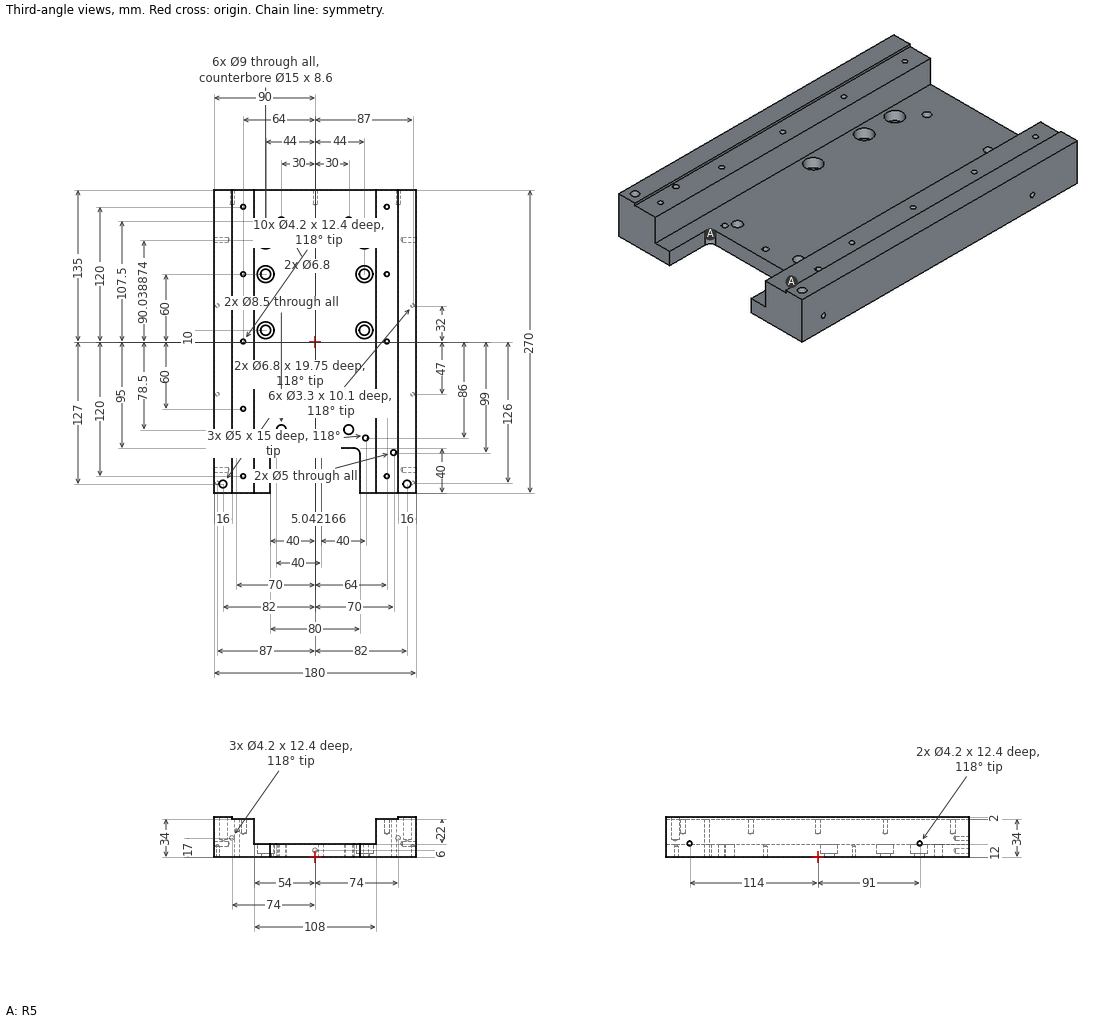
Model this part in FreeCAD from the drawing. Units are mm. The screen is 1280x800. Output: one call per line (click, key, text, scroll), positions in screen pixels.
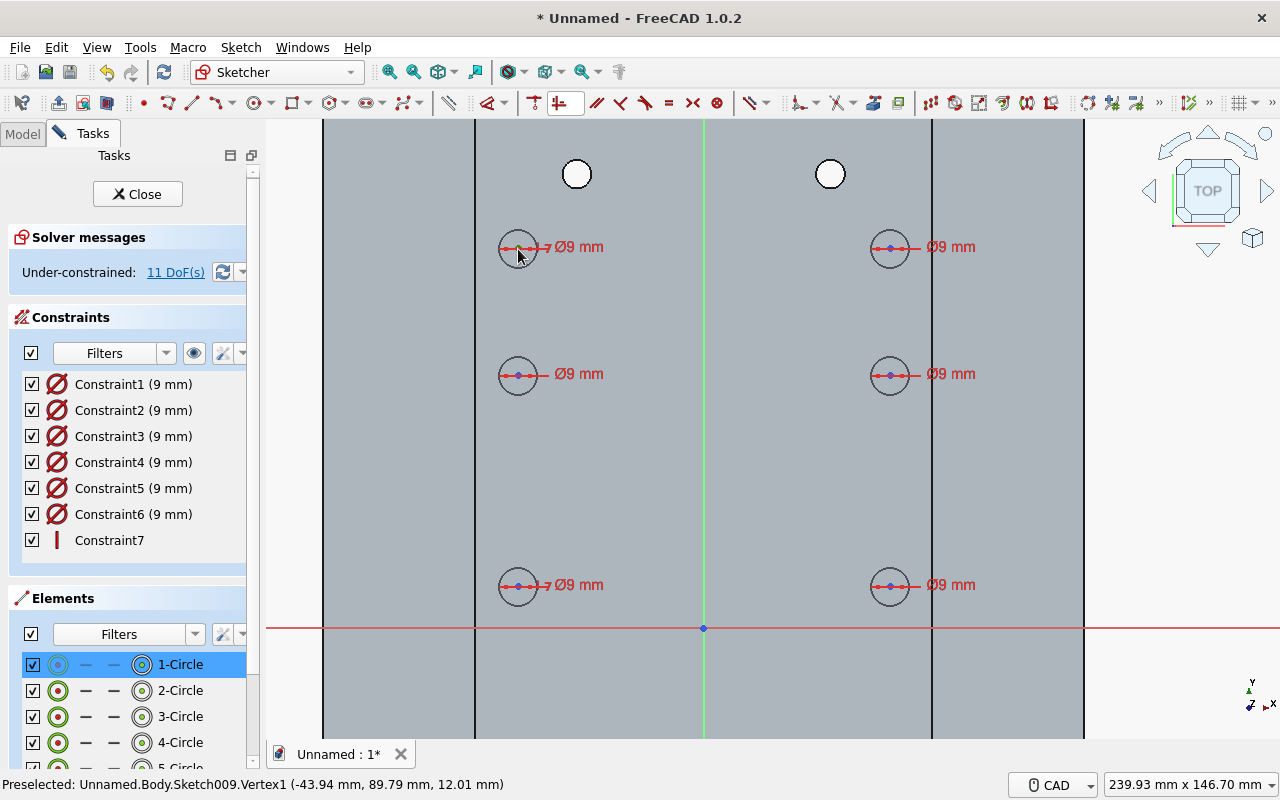
click(518, 376)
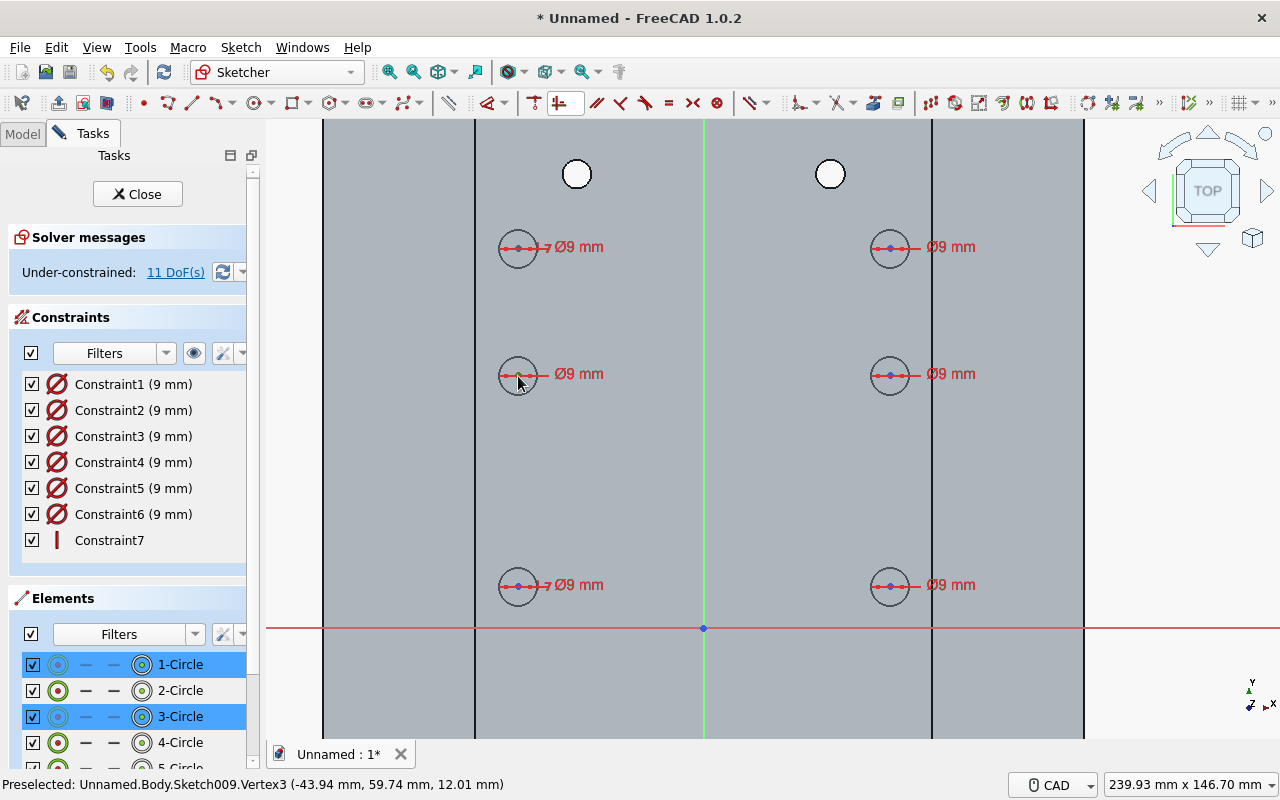
key(v)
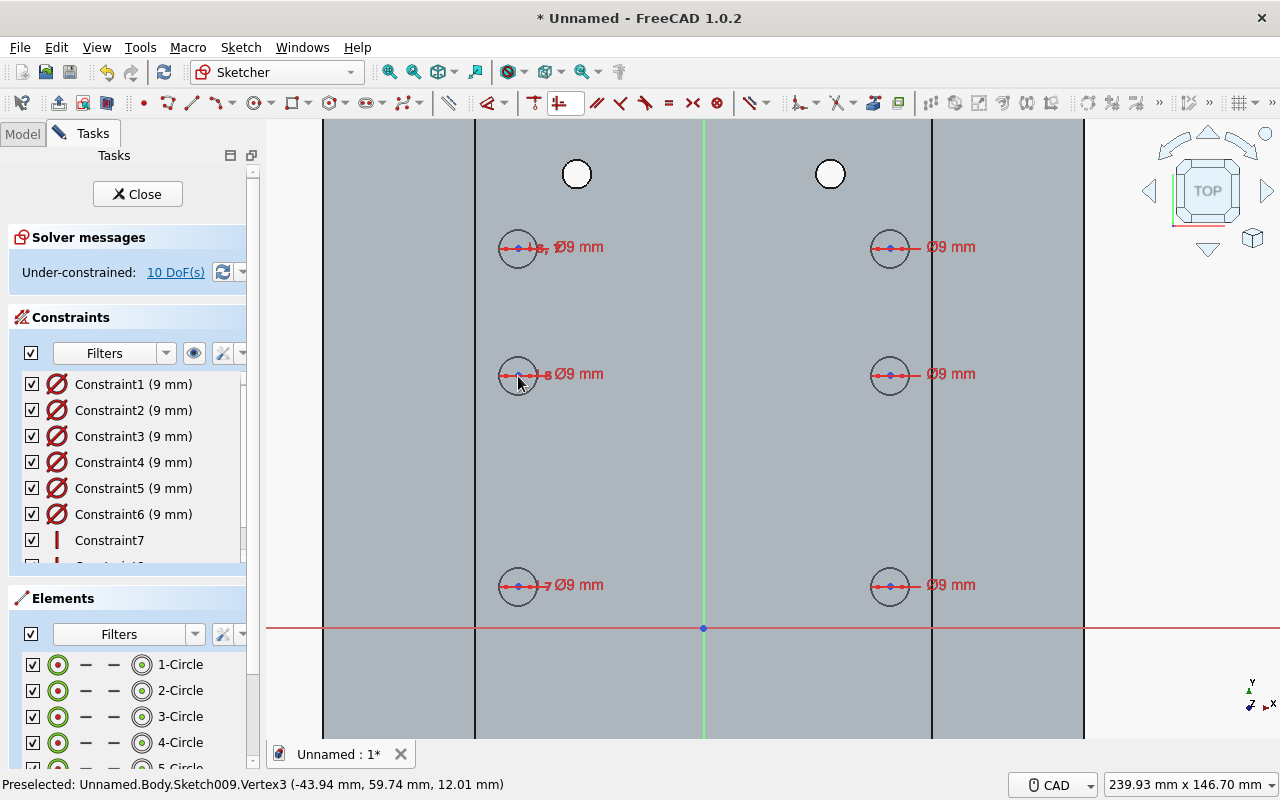
click(518, 376)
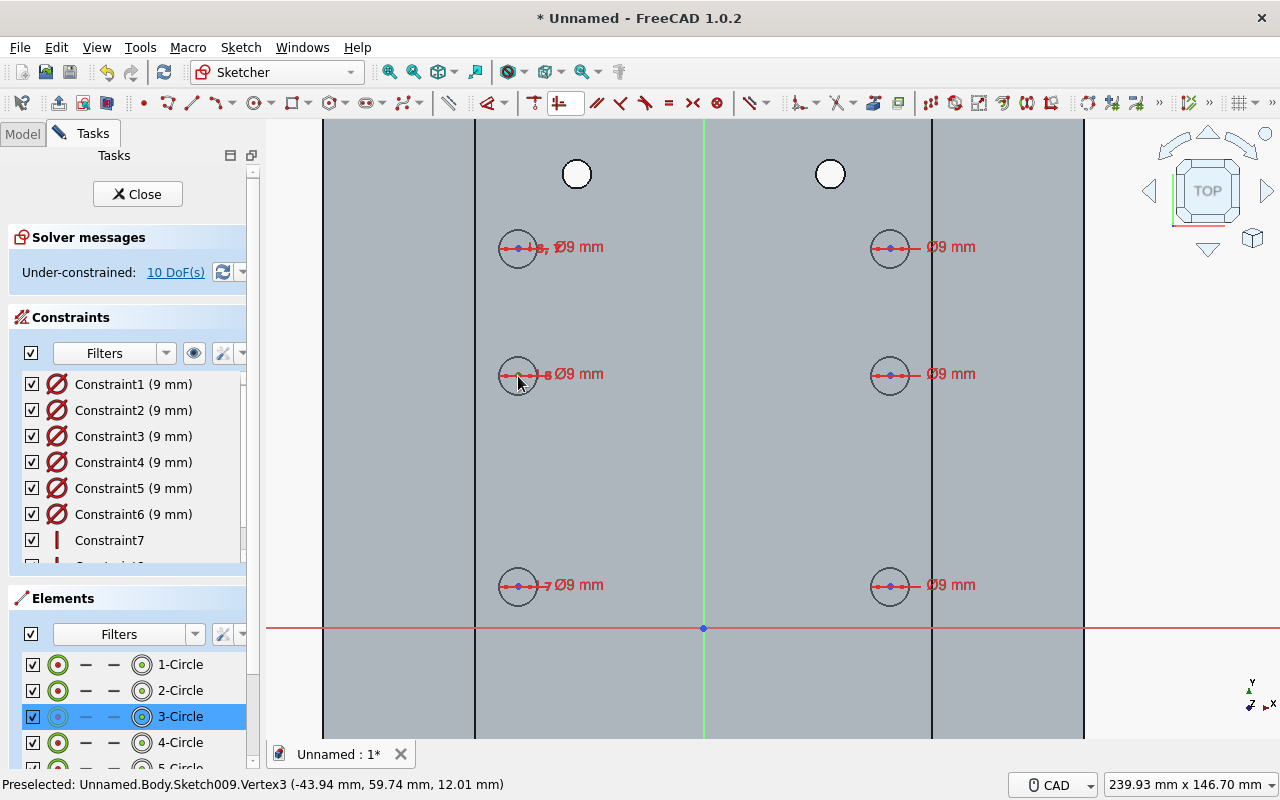
click(890, 376)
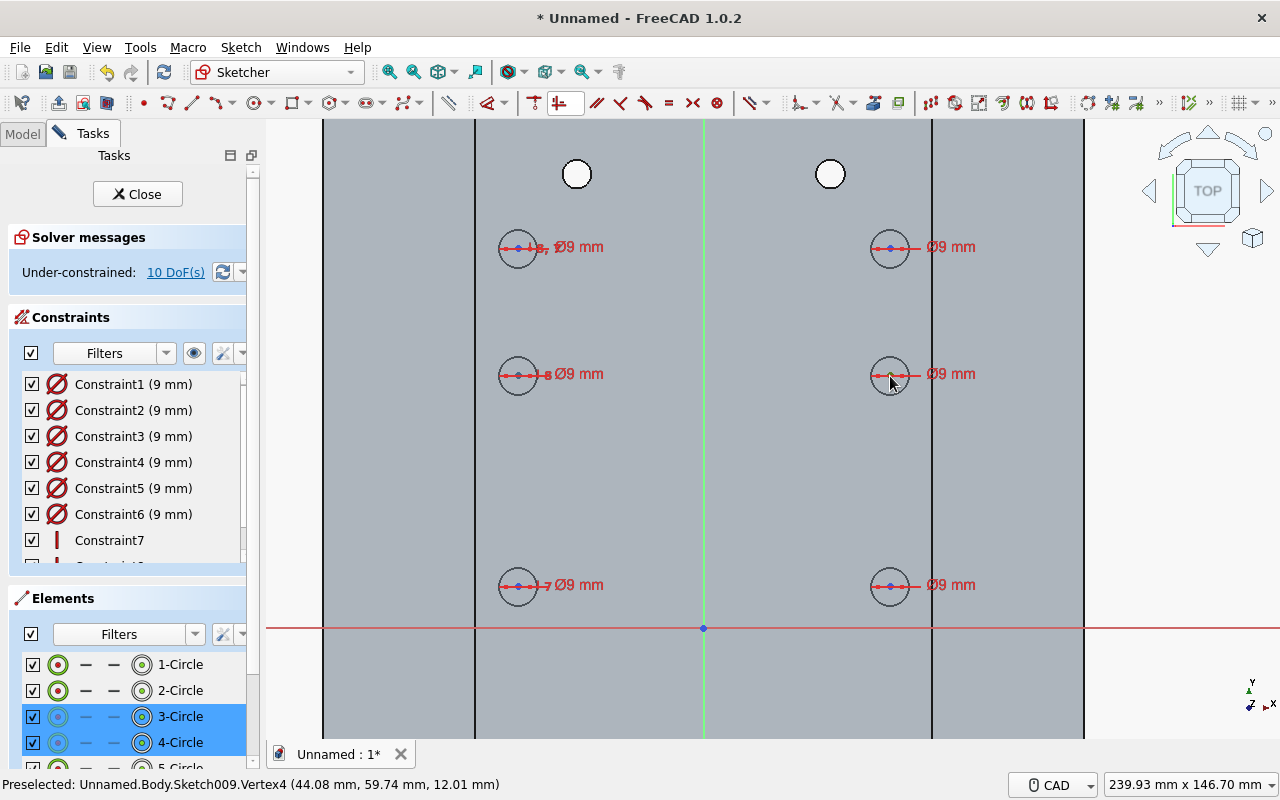
click(578, 104)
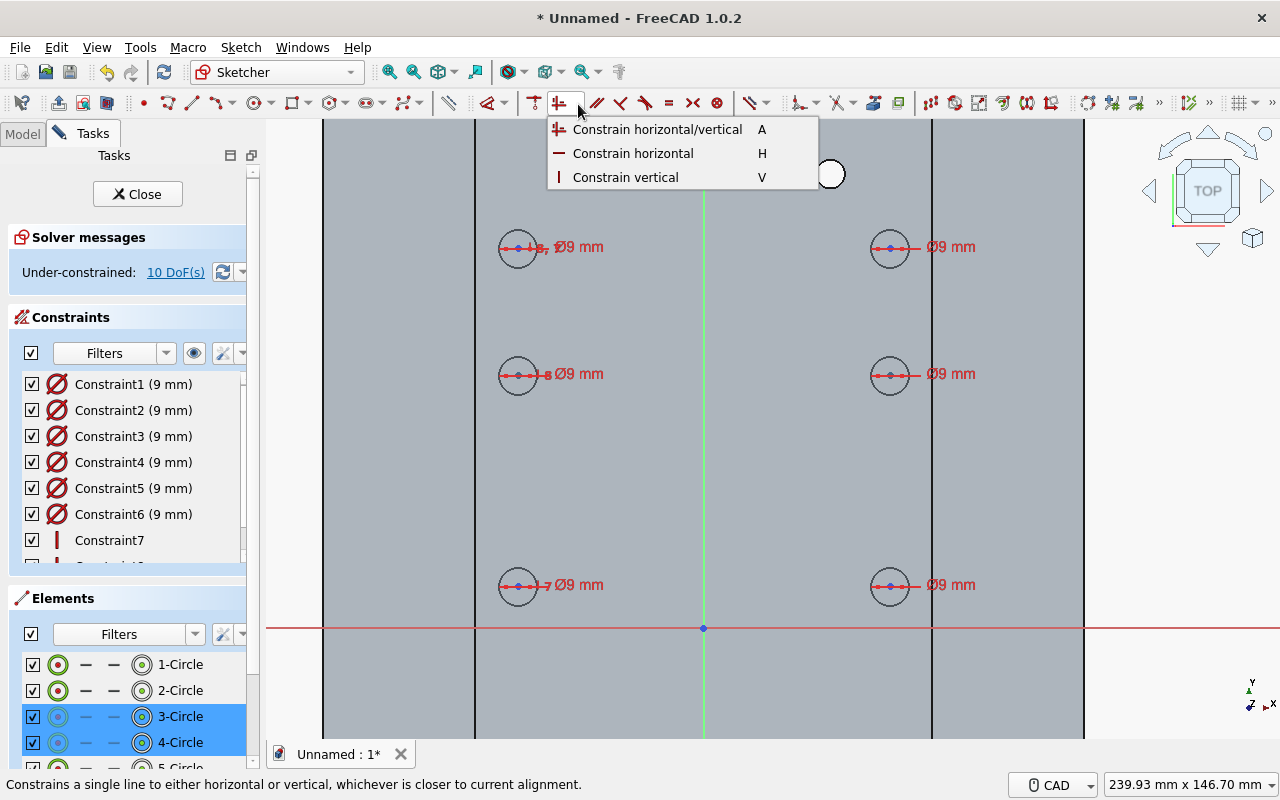
click(683, 153)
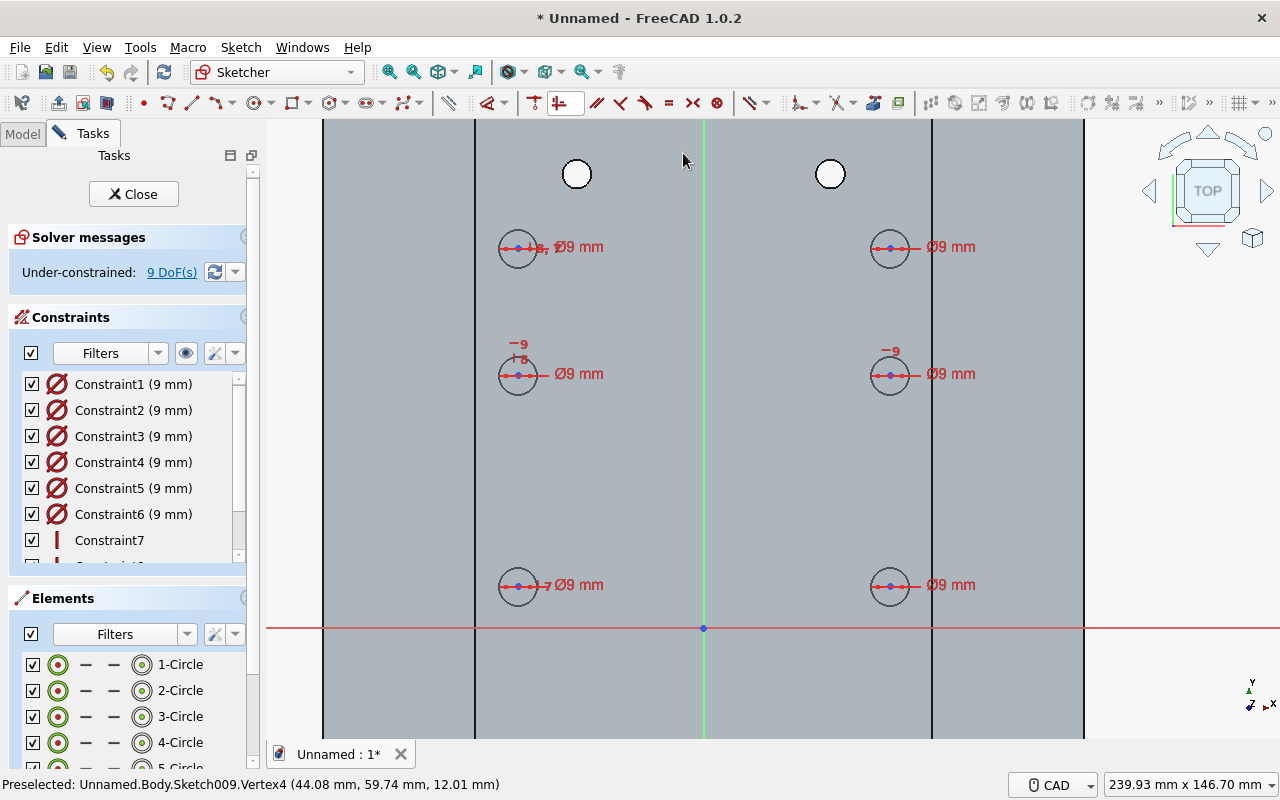
click(890, 376)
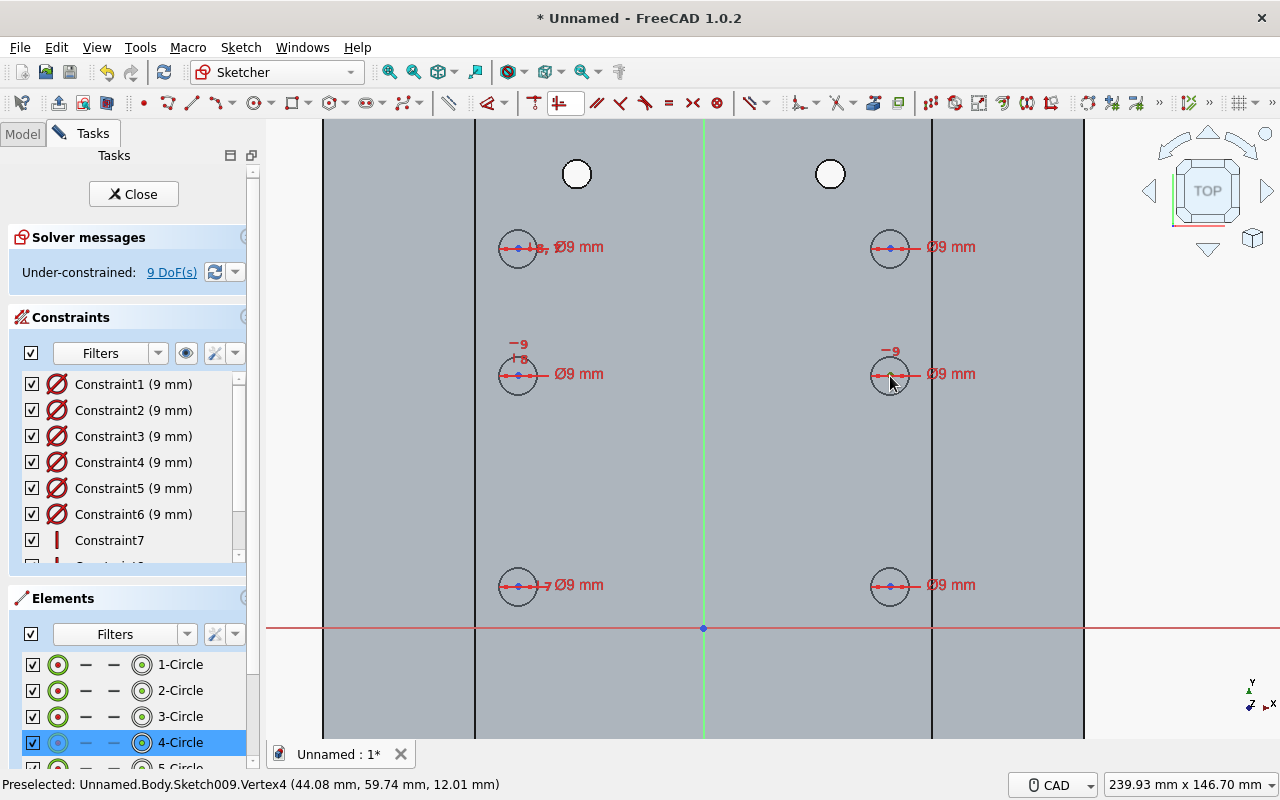
click(890, 587)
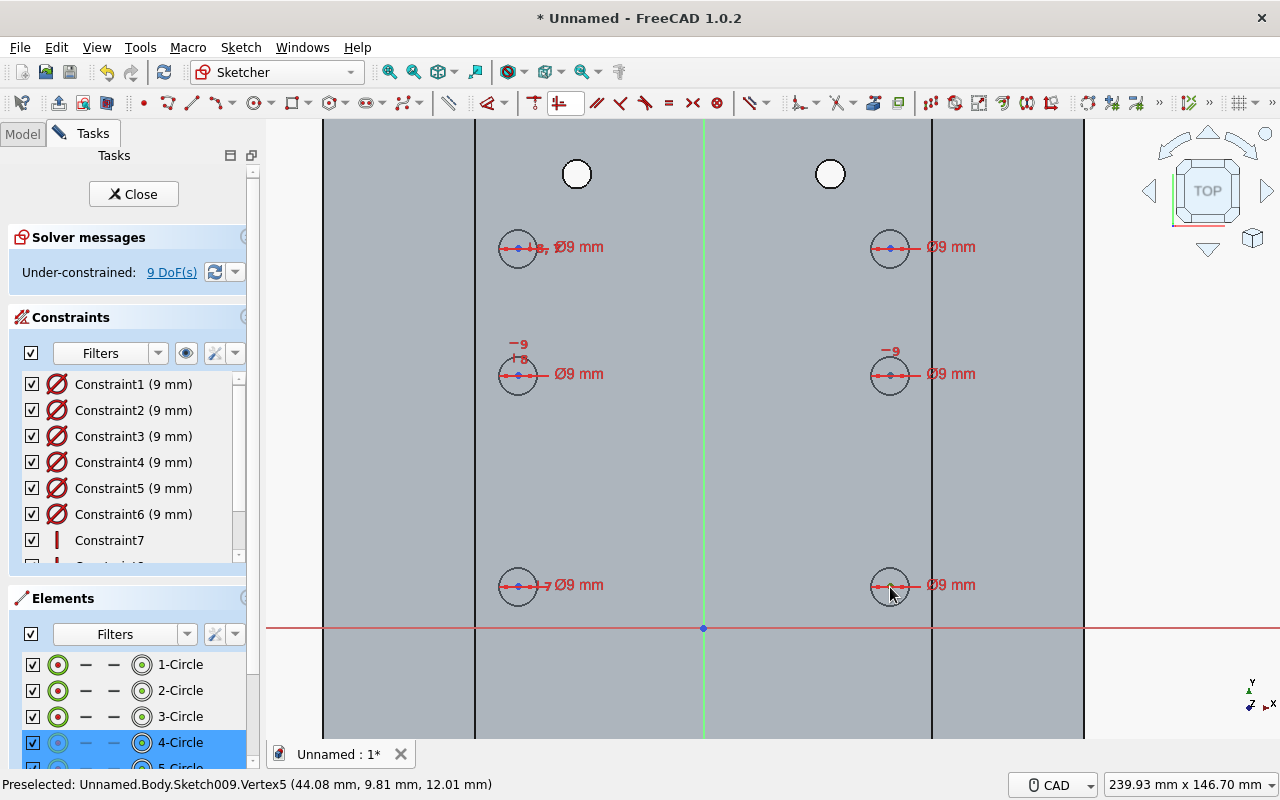
click(578, 104)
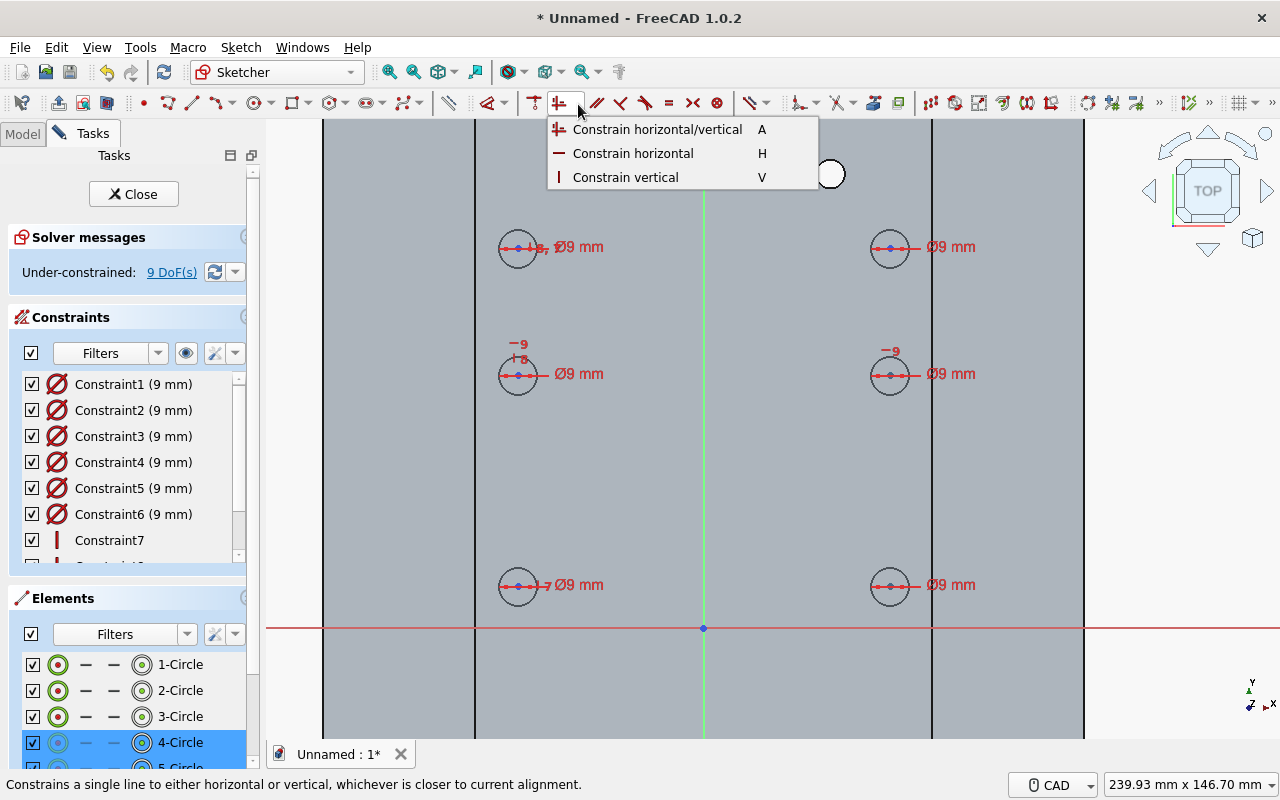
click(683, 177)